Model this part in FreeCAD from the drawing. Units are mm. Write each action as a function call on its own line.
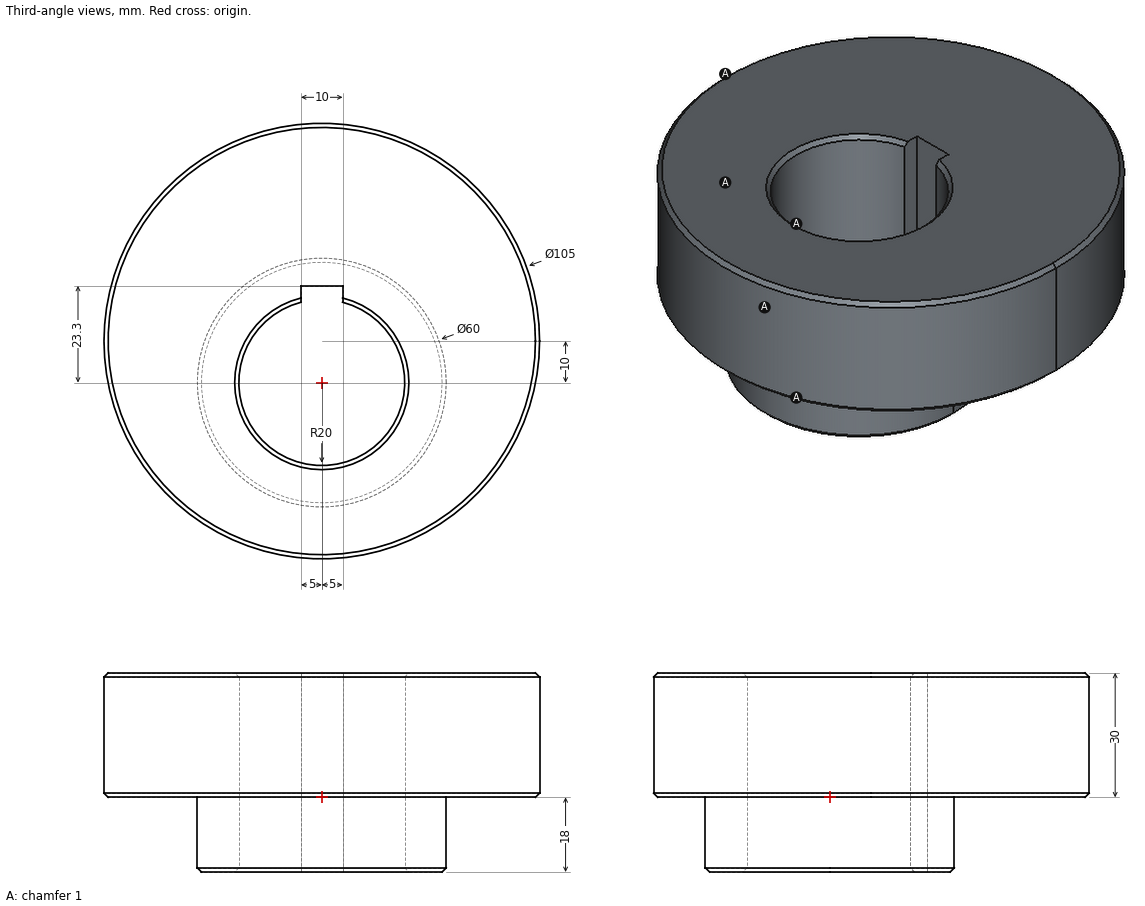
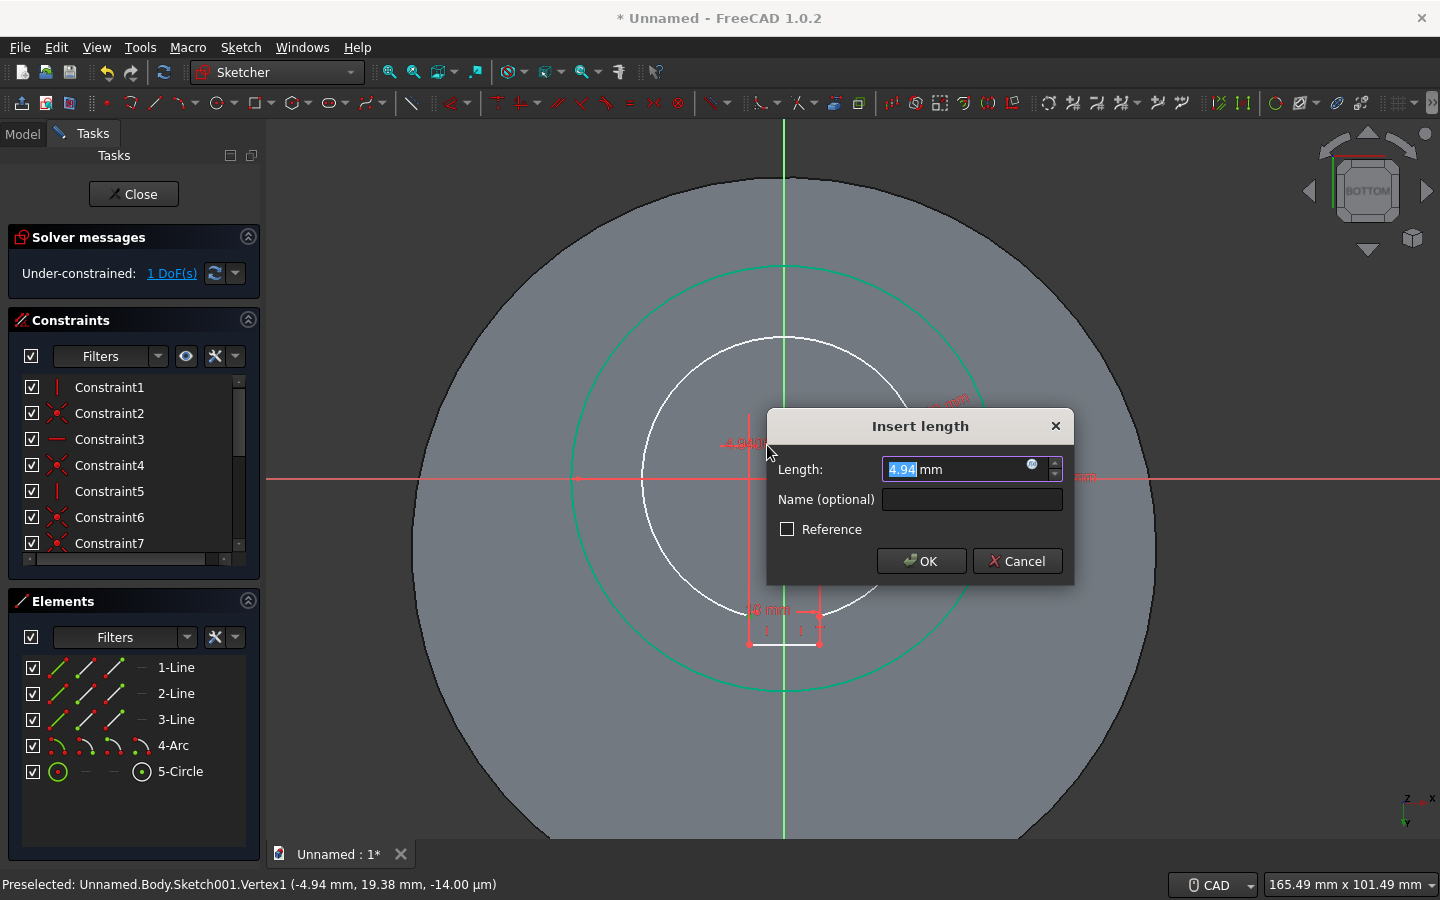
text(5)
key(Return)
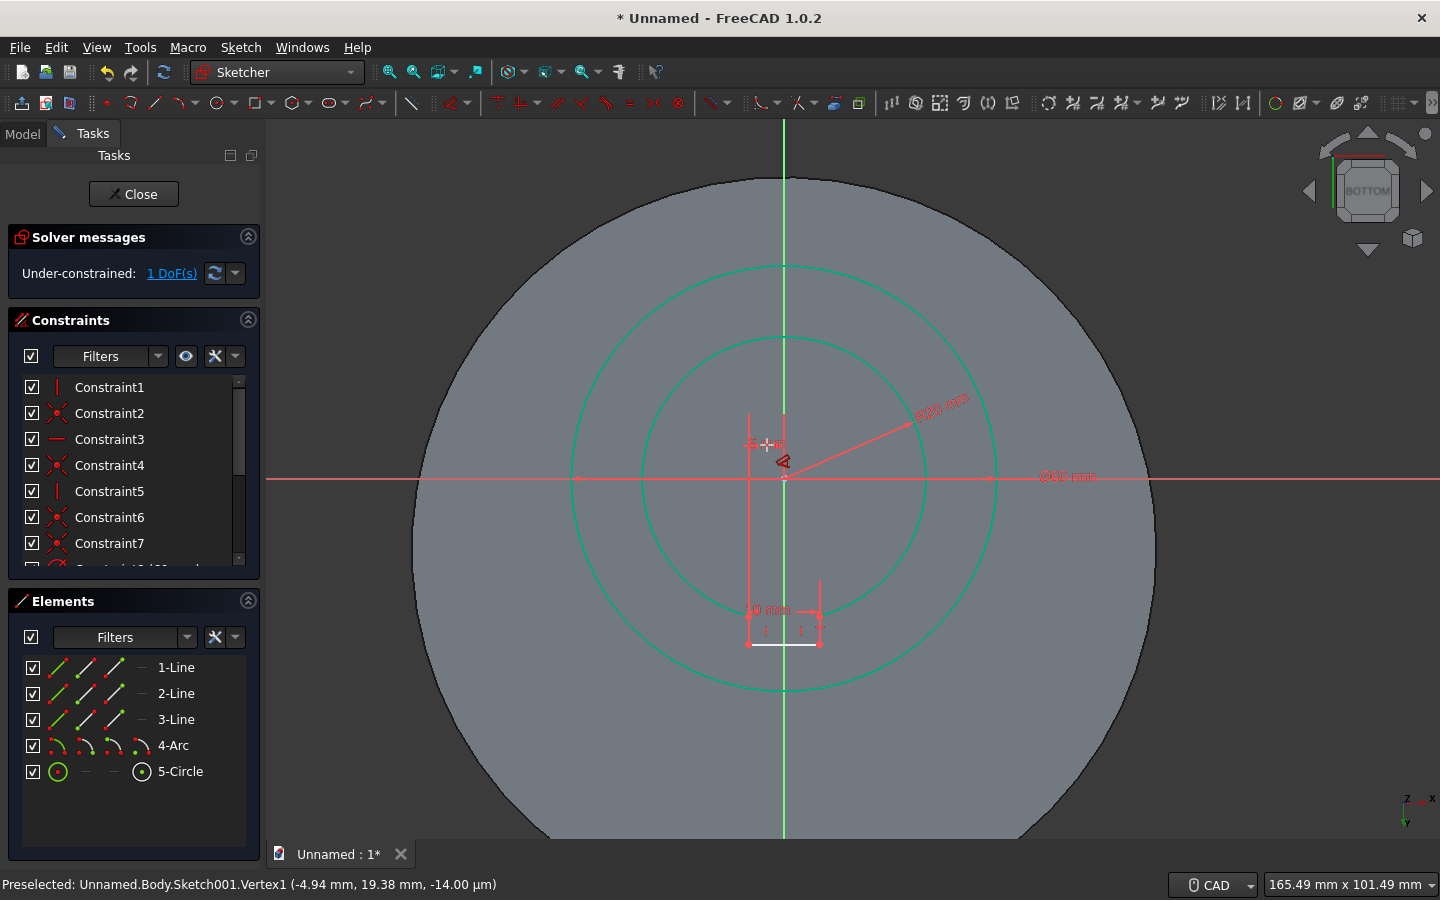
click(749, 645)
click(715, 562)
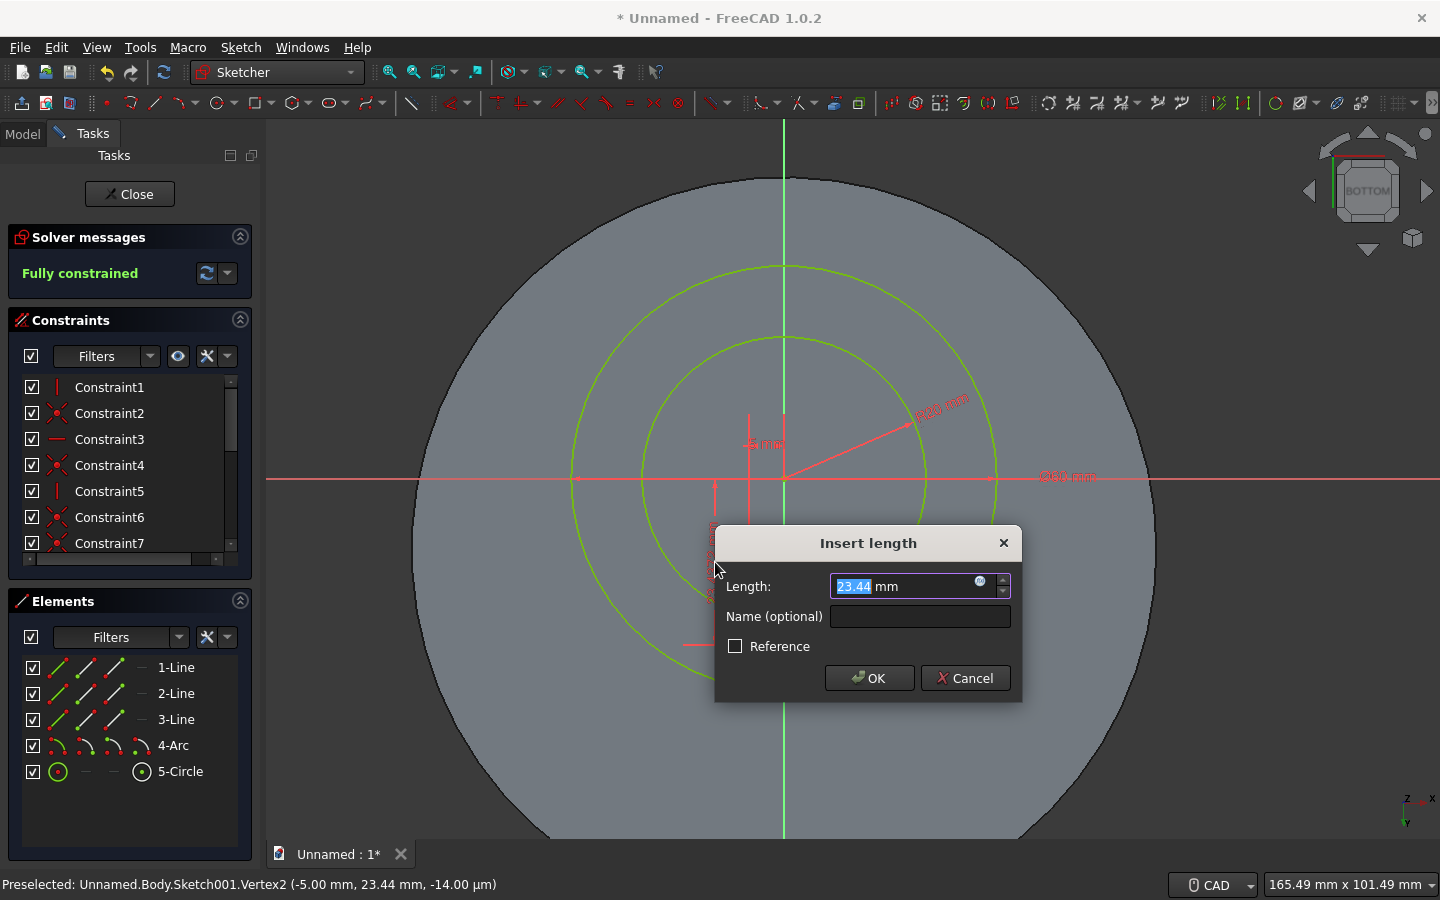
text(23.3)
key(Return)
key(Escape)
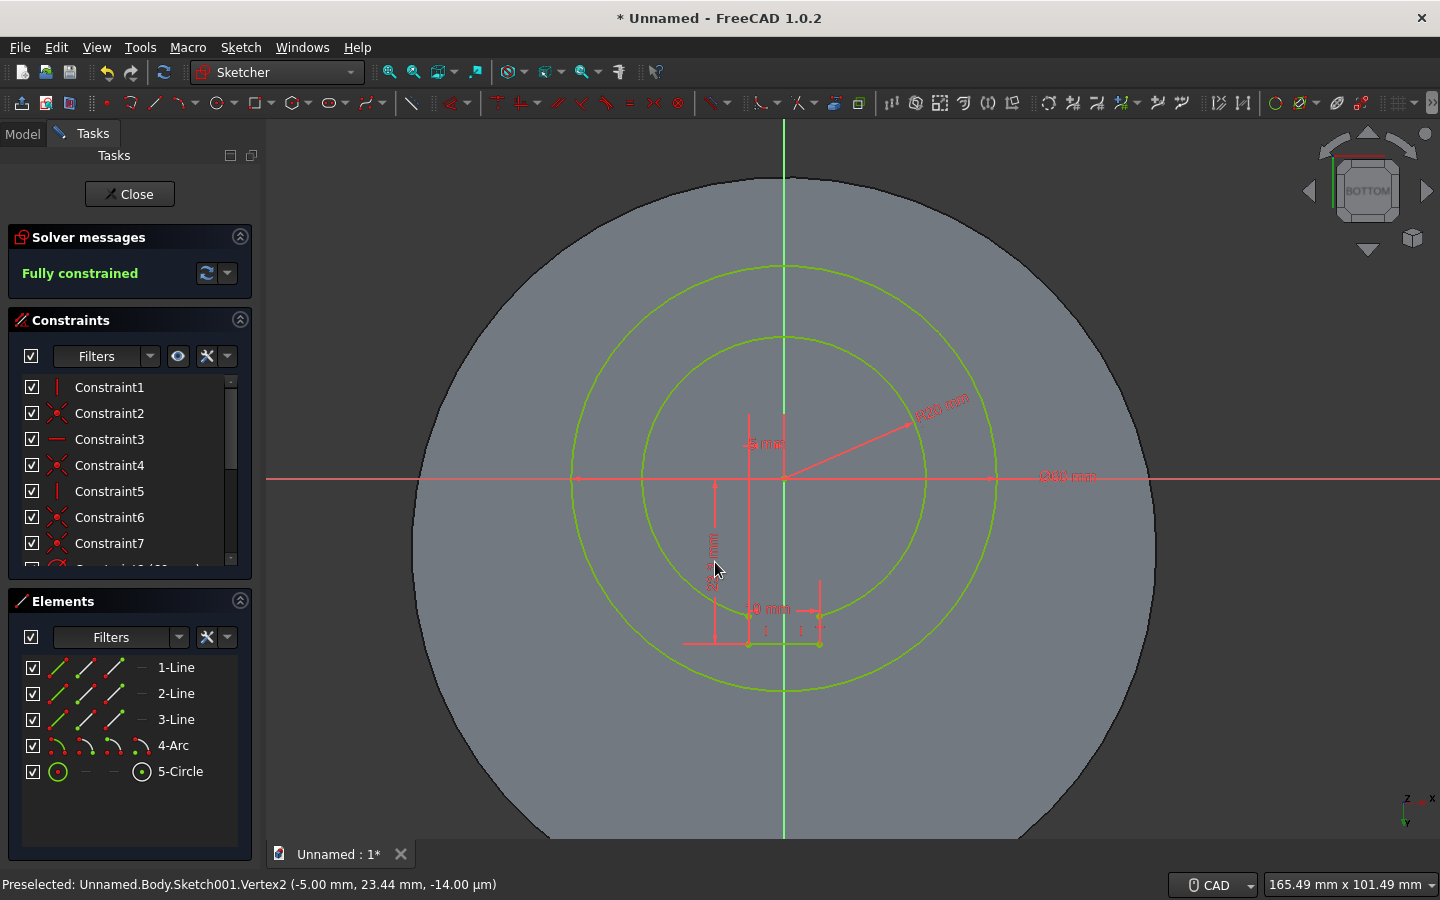
click(130, 194)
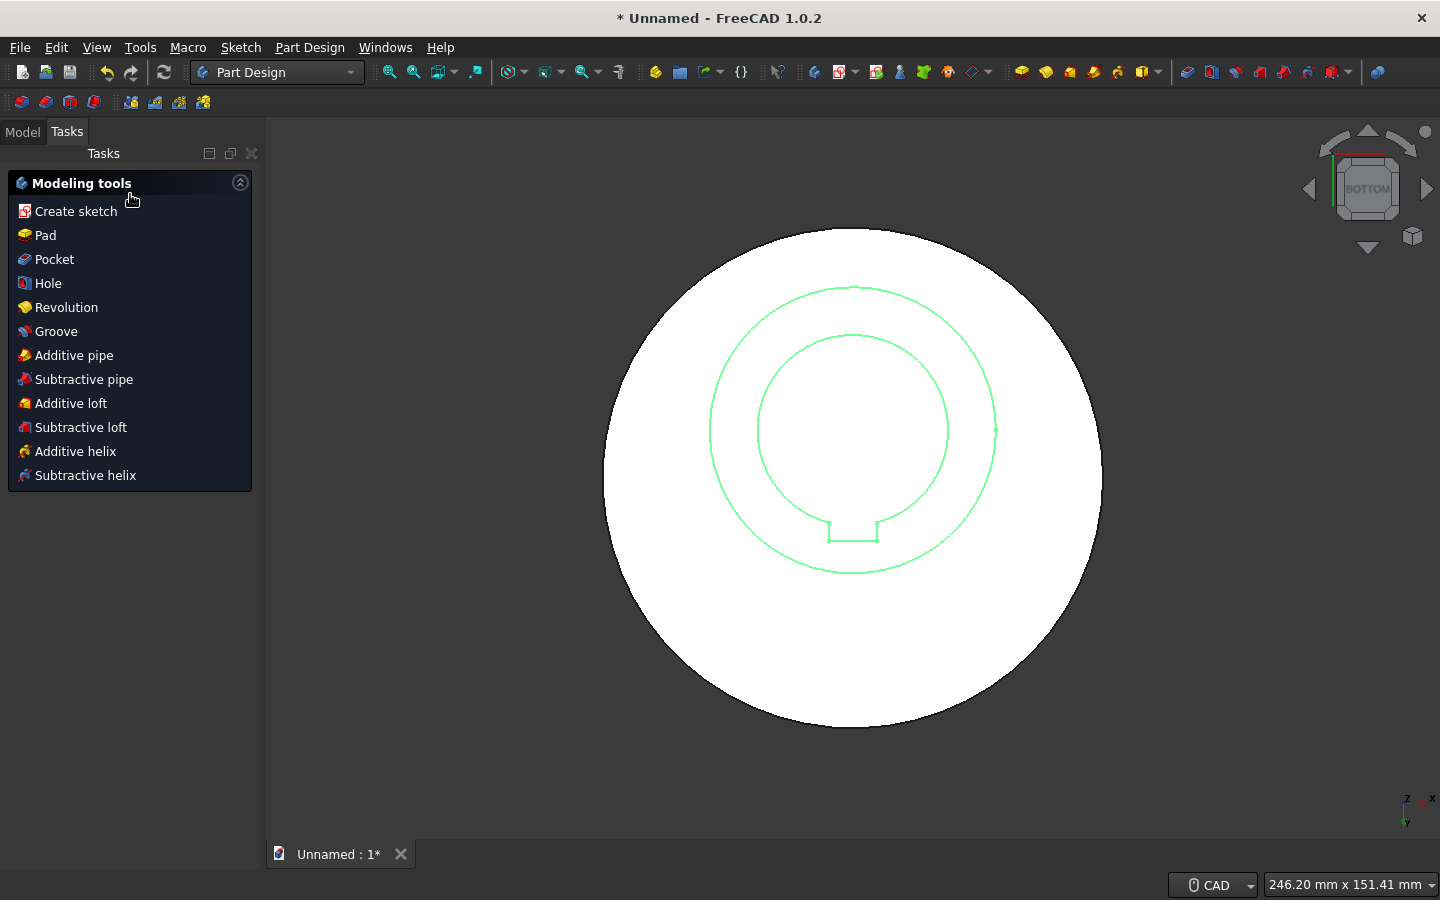
click(1022, 72)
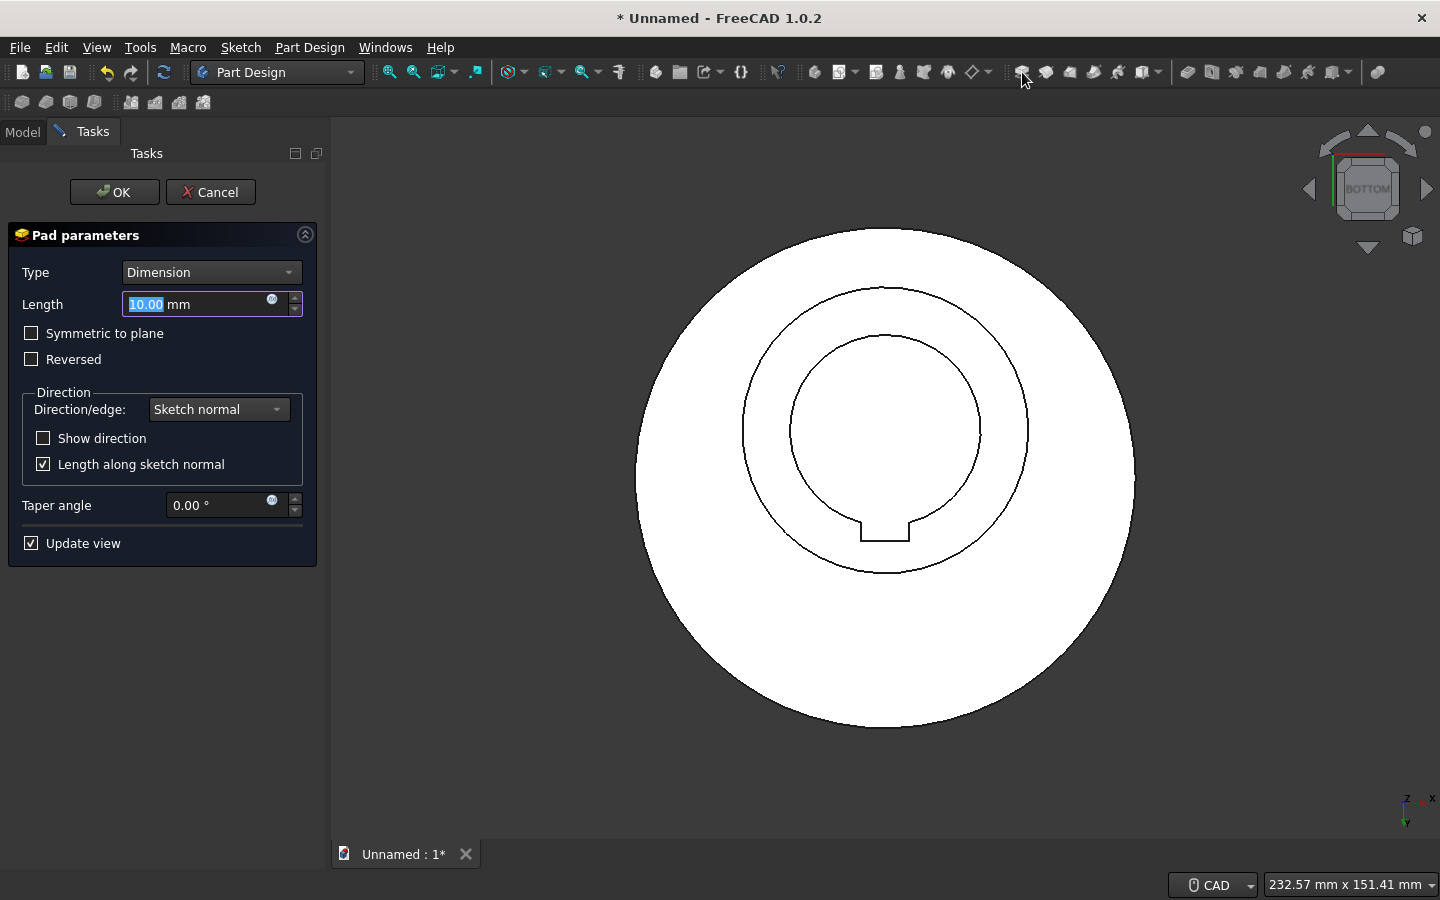
text(18)
key(Tab)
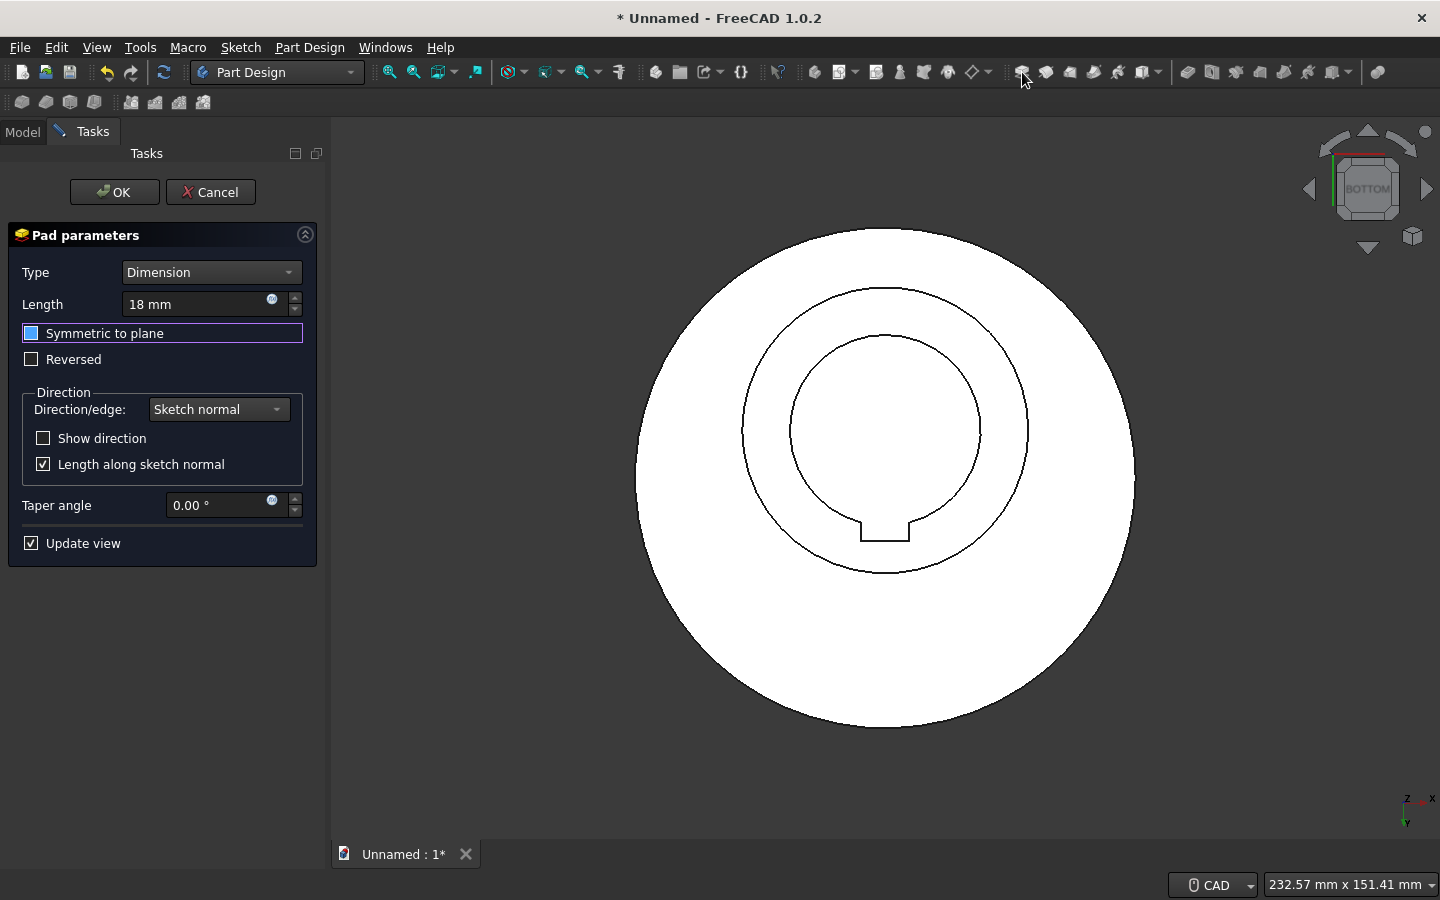
click(115, 192)